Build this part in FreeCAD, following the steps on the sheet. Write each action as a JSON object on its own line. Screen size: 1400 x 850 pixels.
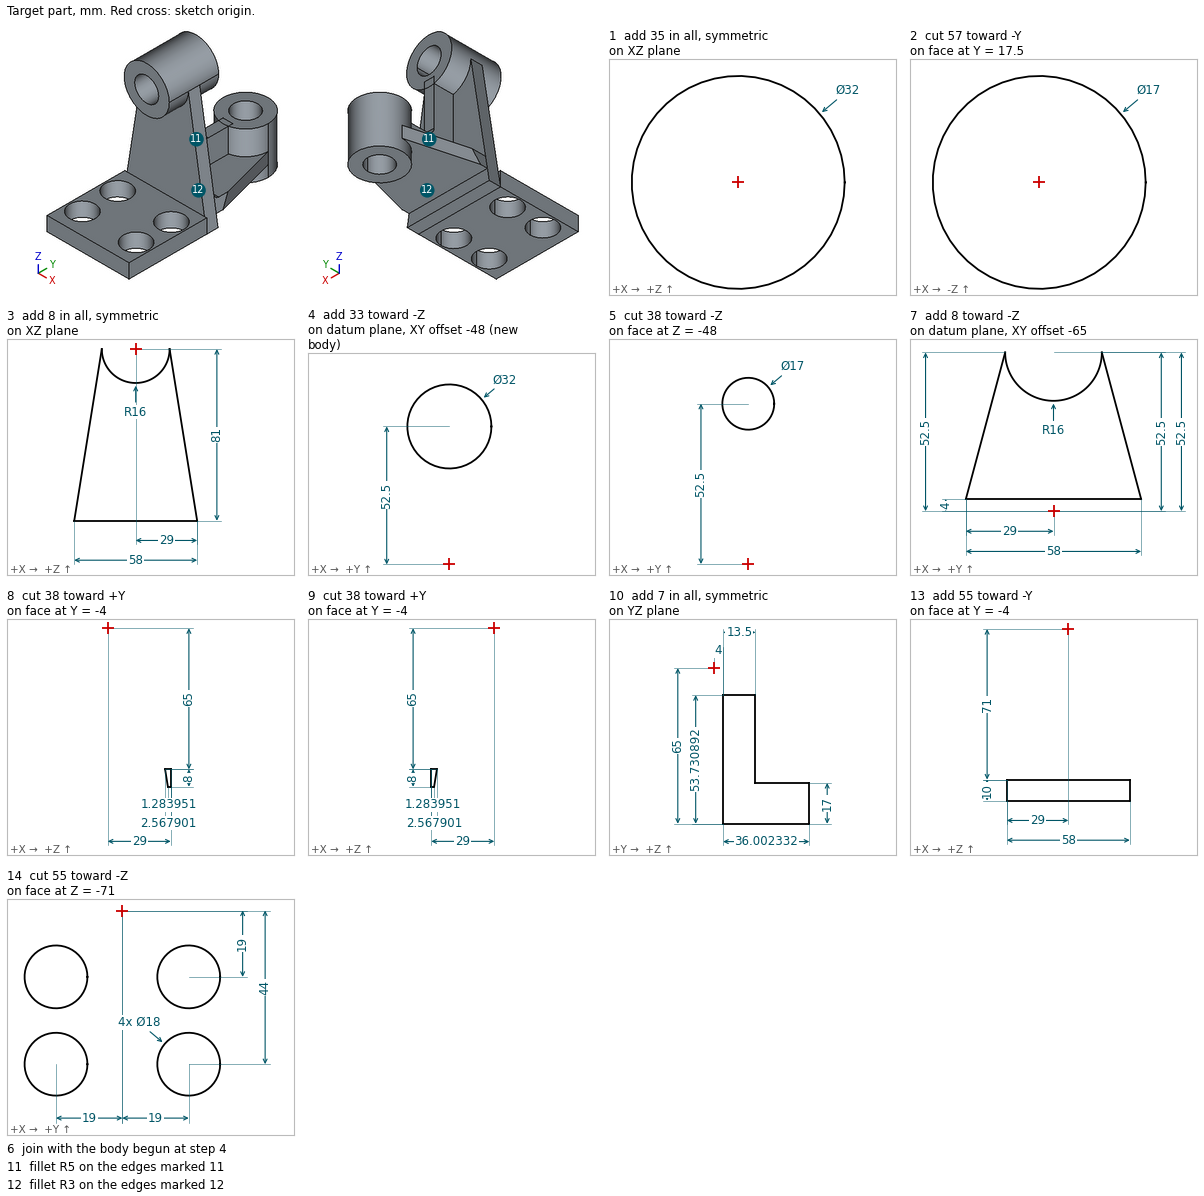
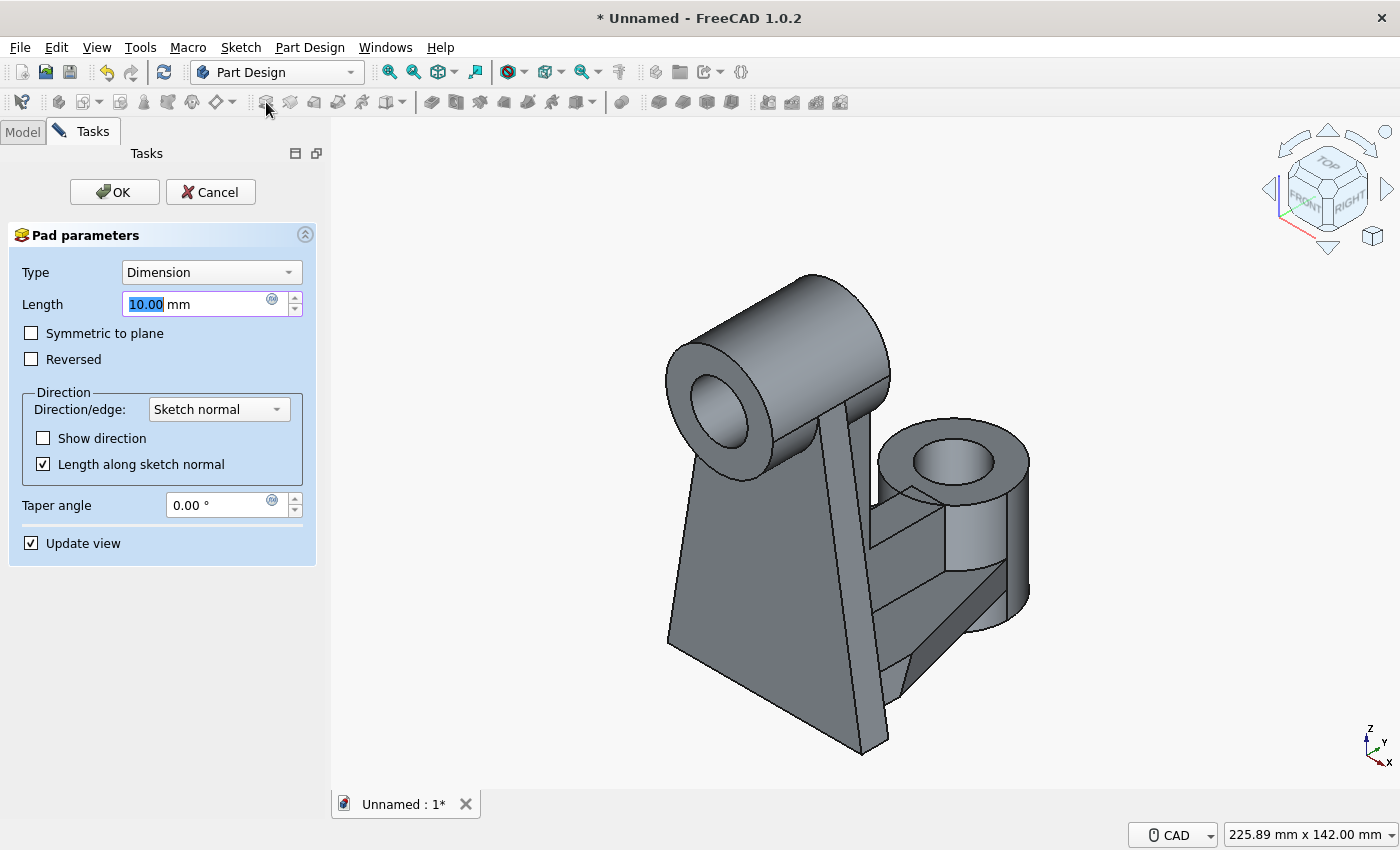
{"action": "type", "text": "7"}
{"action": "key", "text": "Tab"}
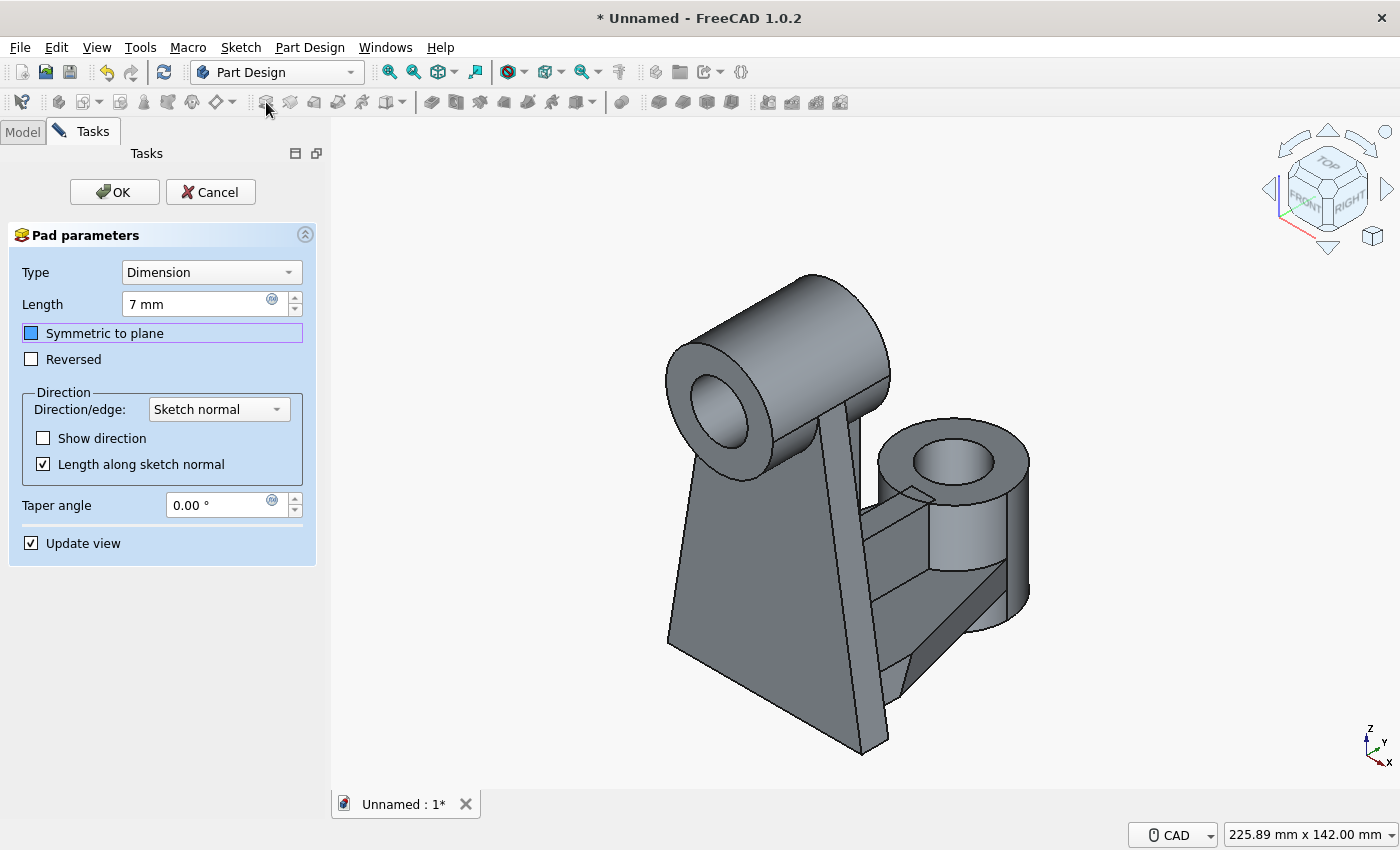
{"action": "left_click", "coordinate": [30, 333]}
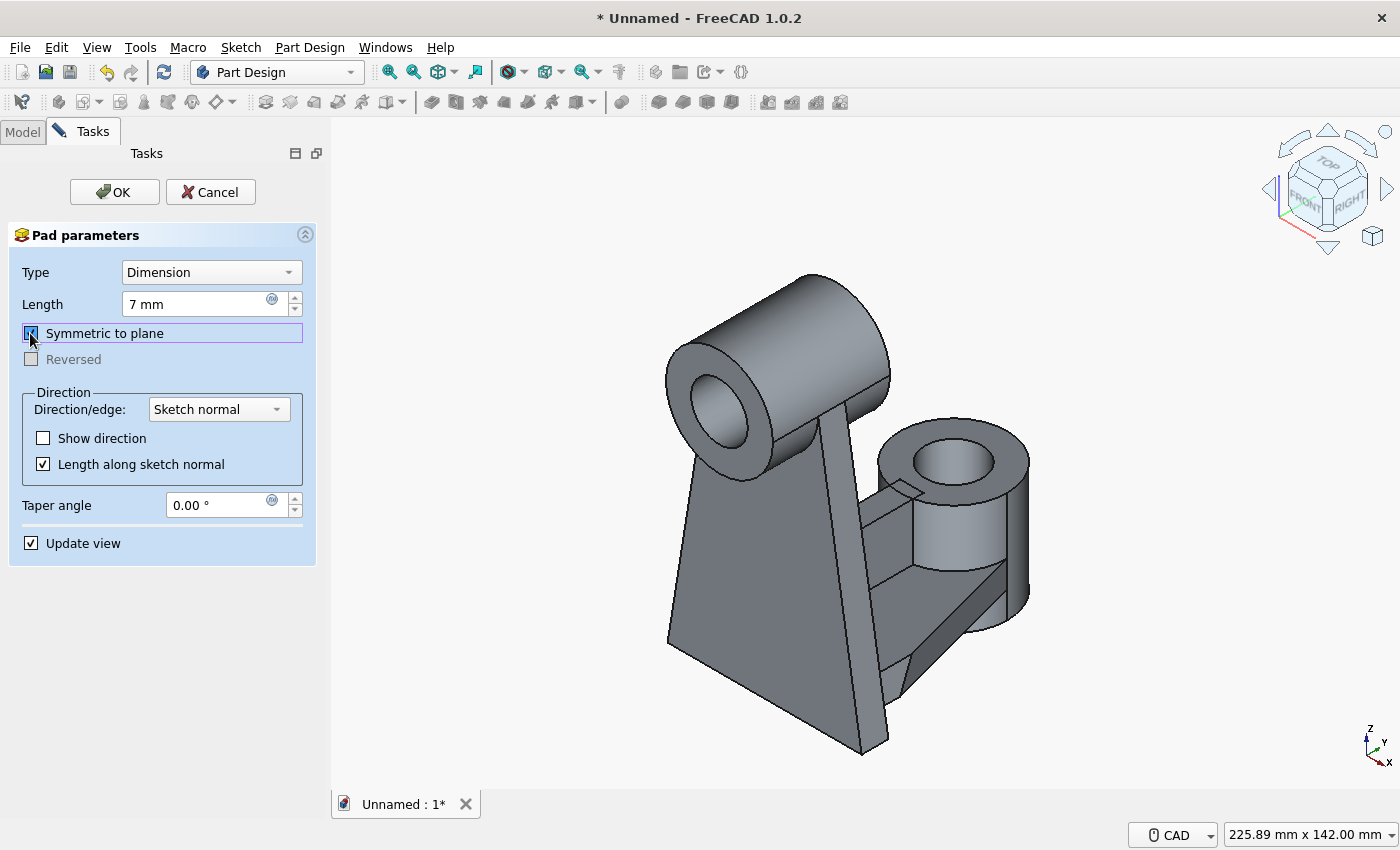
{"action": "left_click", "coordinate": [115, 192]}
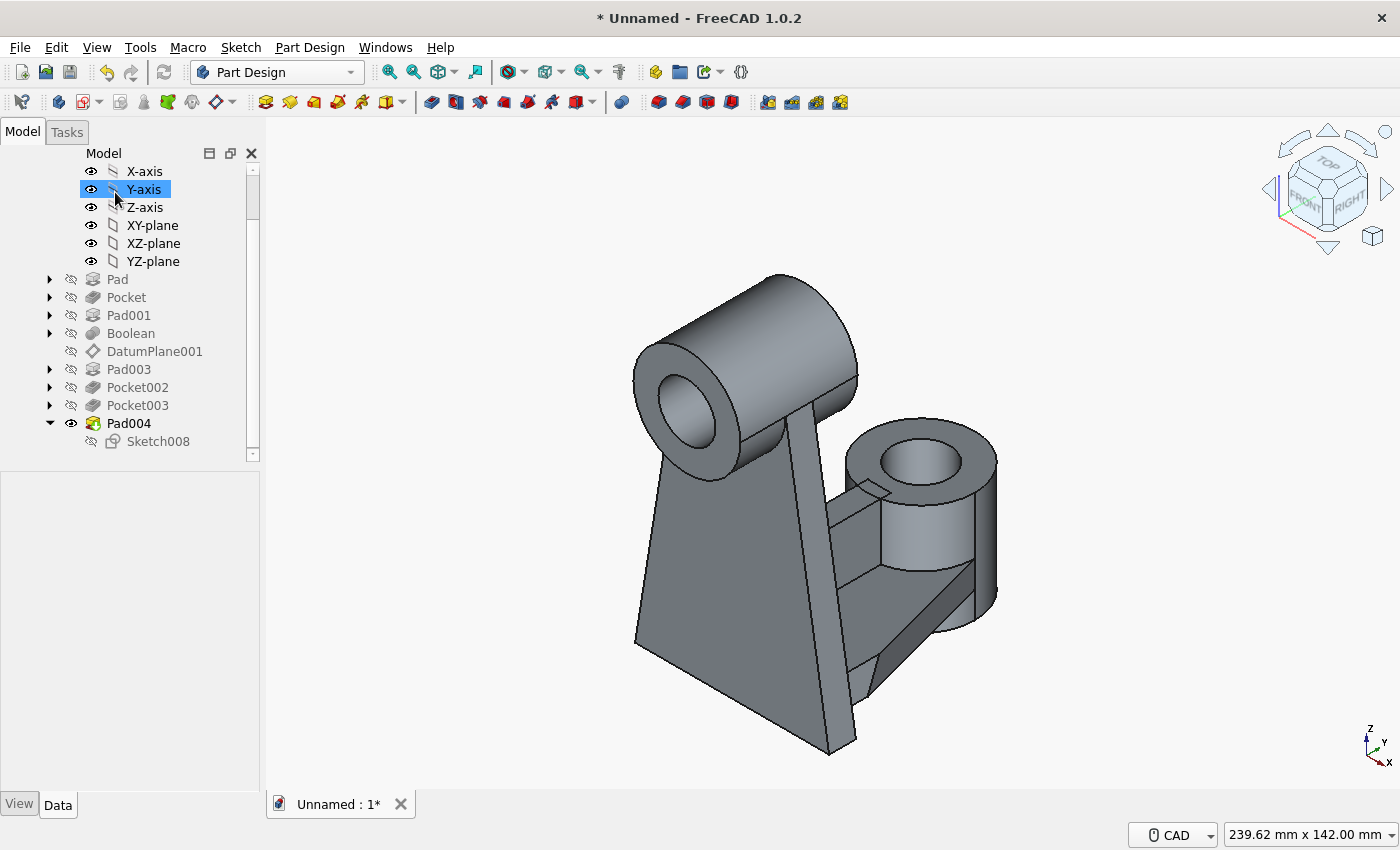
{"action": "key", "text": "2"}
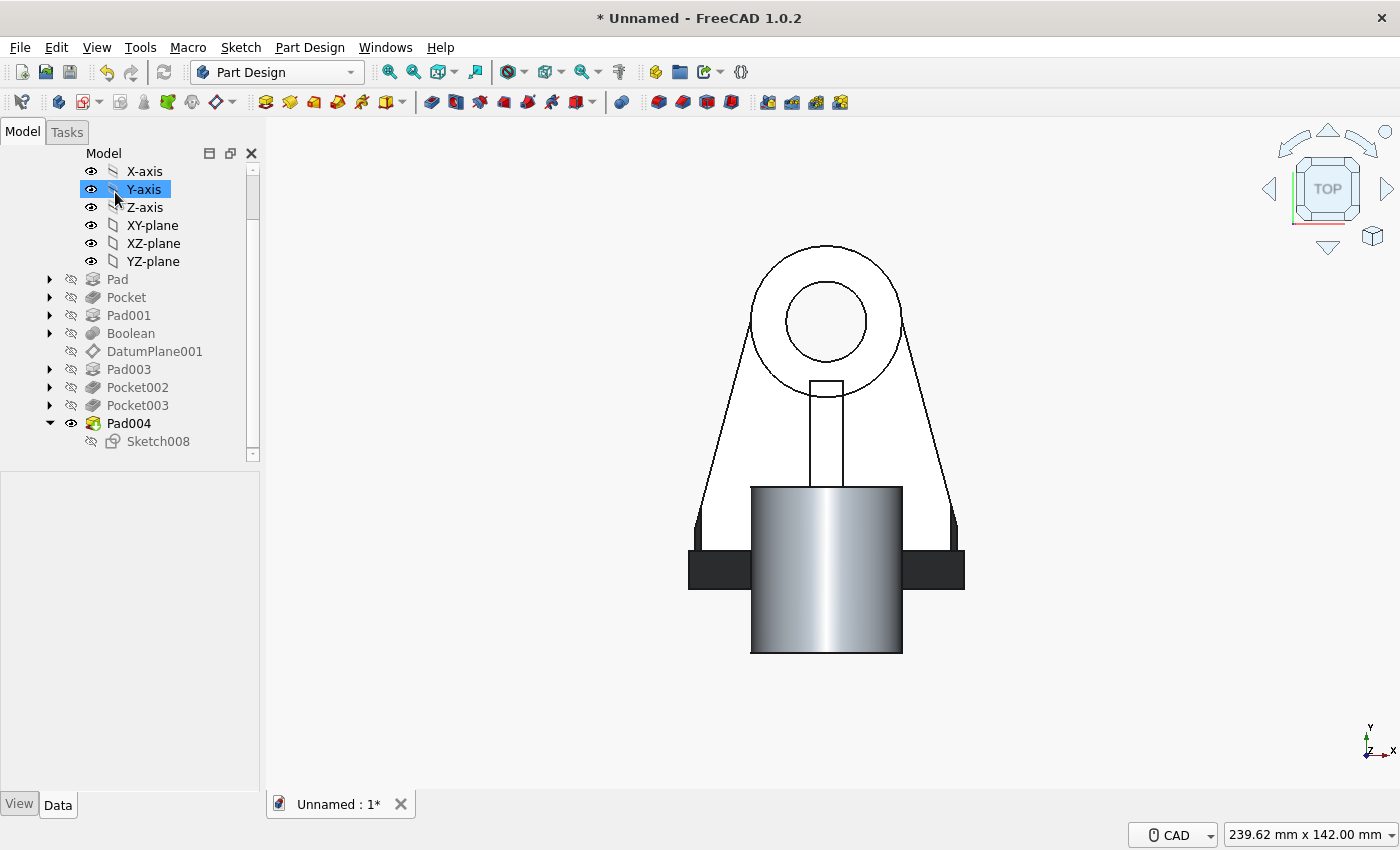
{"action": "key", "text": "0"}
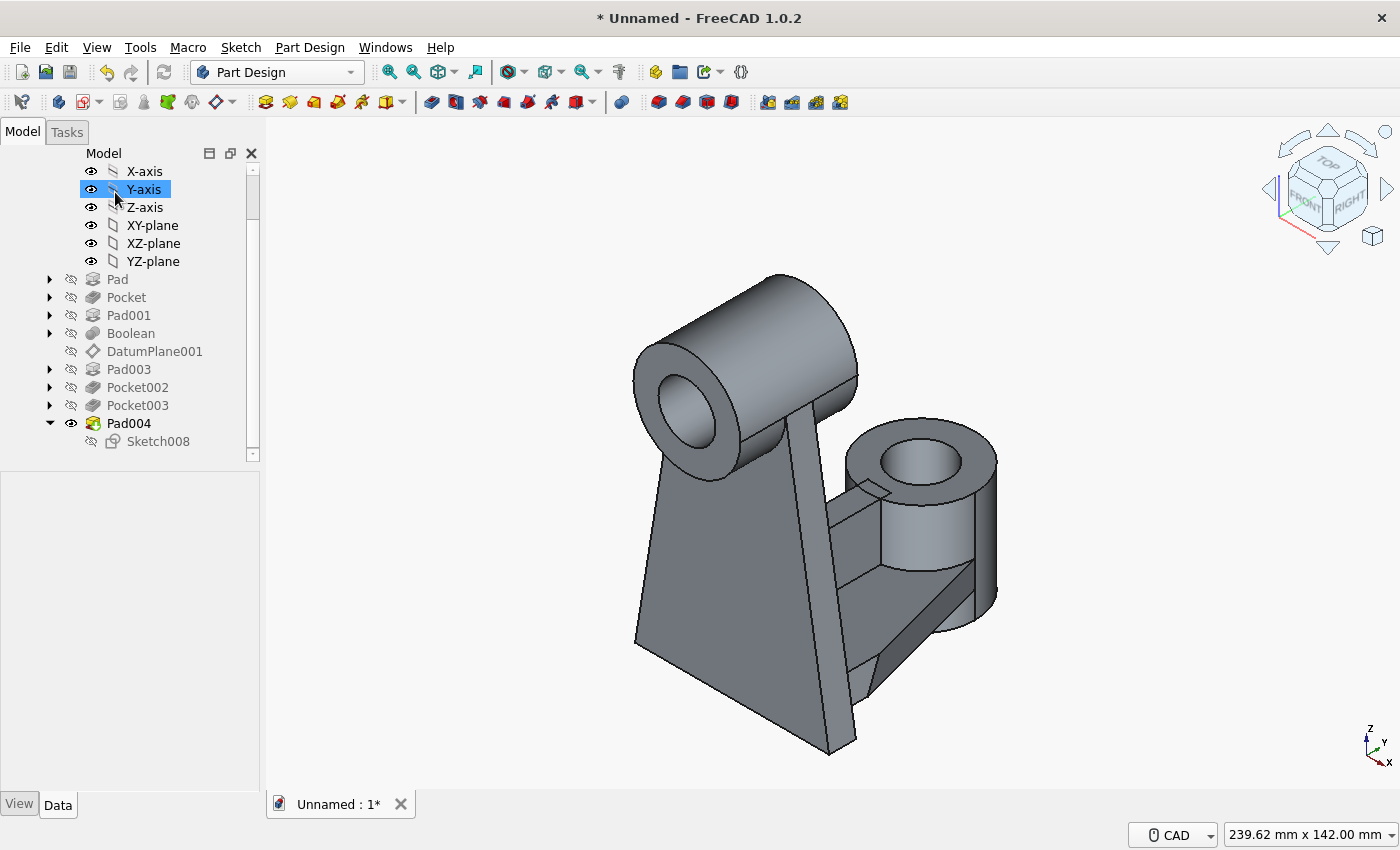
{"action": "key", "text": "1"}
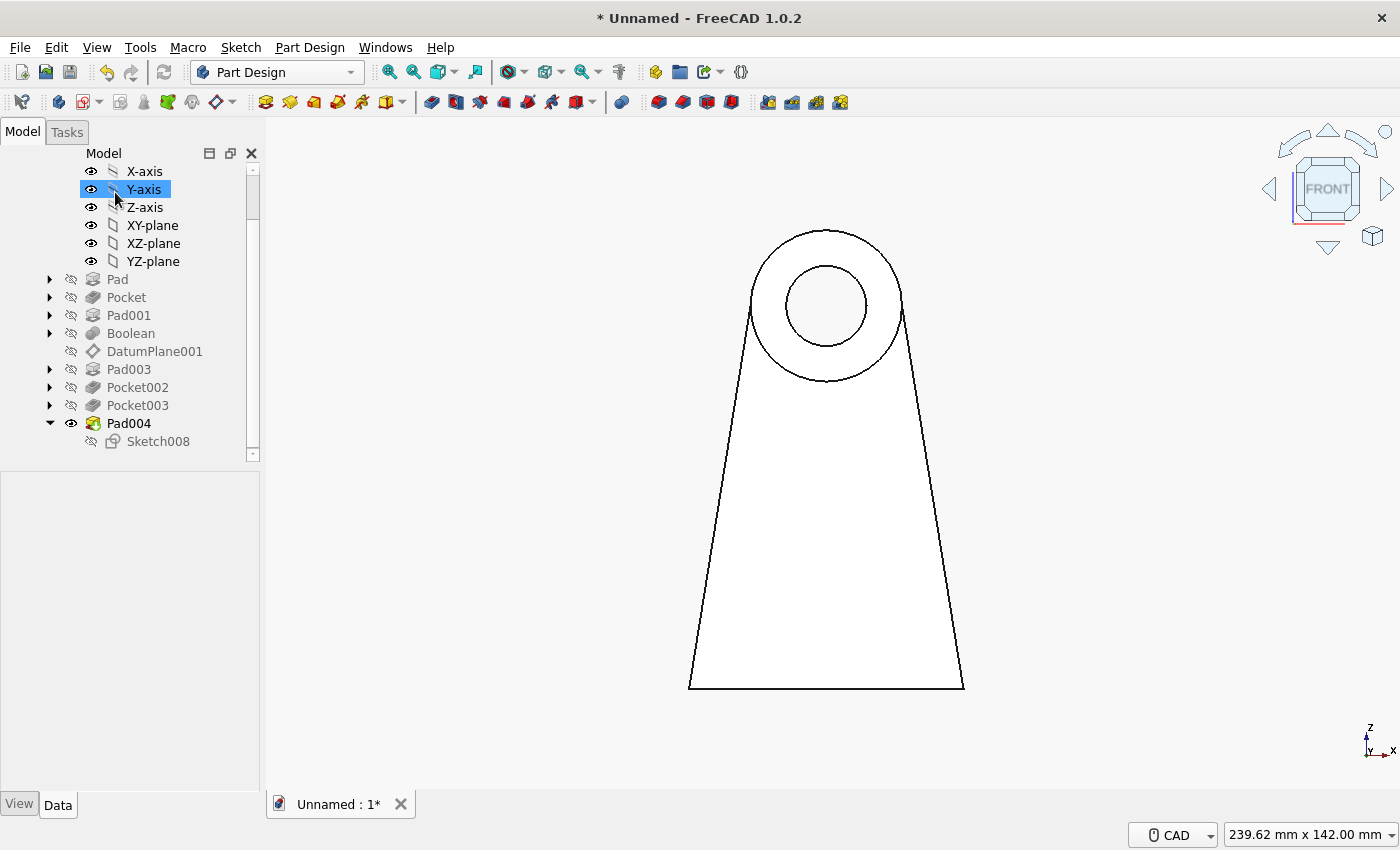
{"action": "key", "text": "3"}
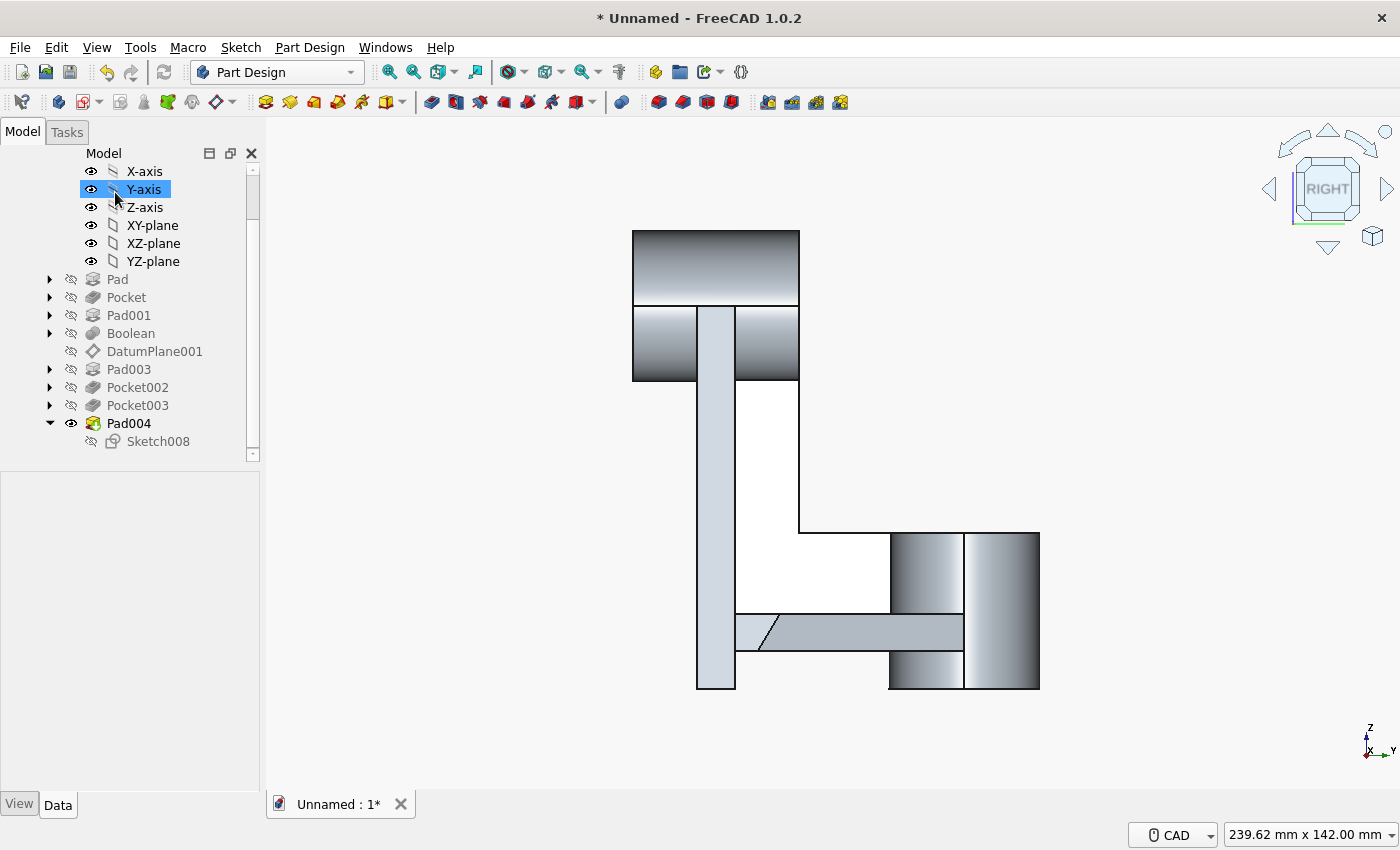
{"action": "key", "text": "5"}